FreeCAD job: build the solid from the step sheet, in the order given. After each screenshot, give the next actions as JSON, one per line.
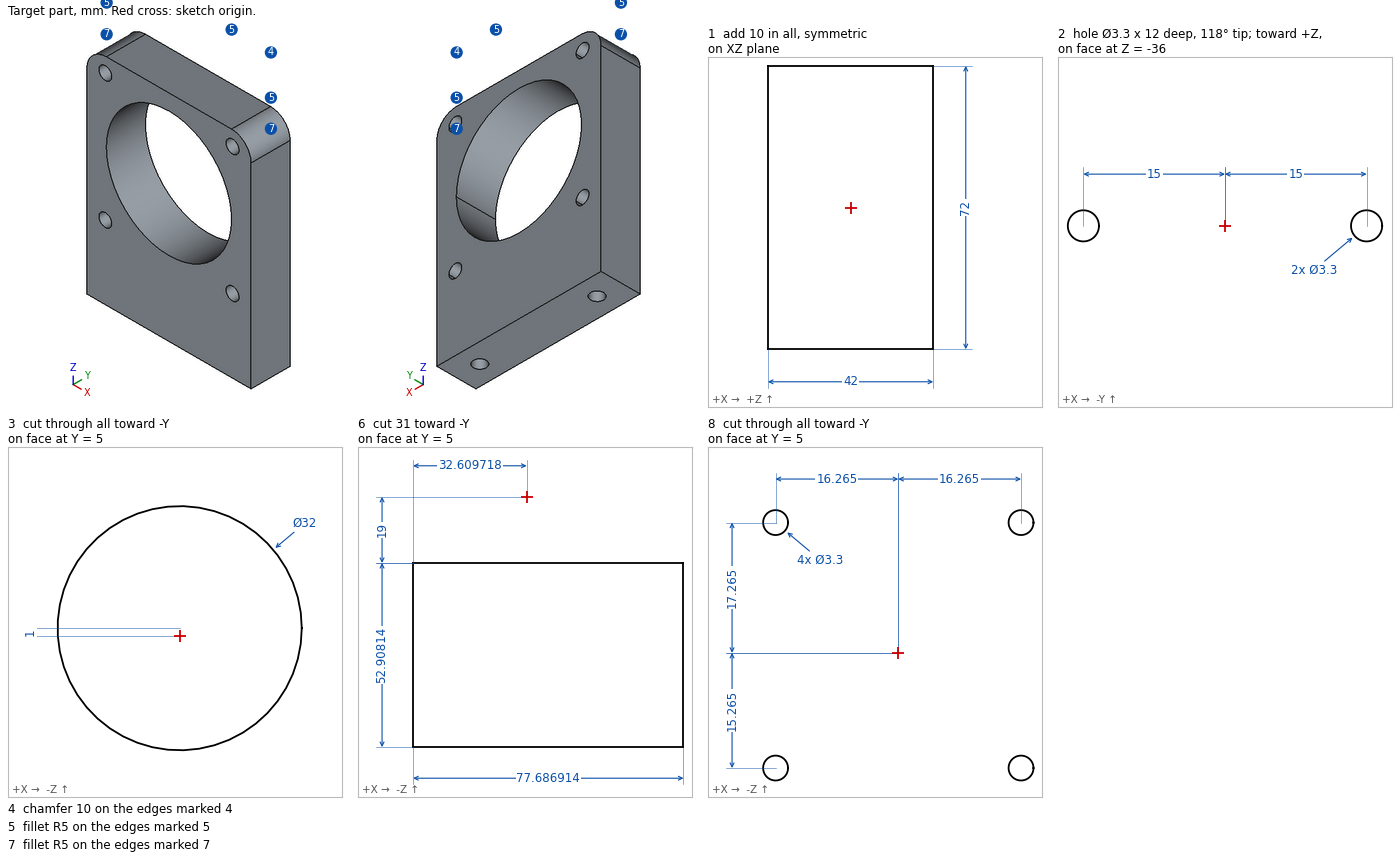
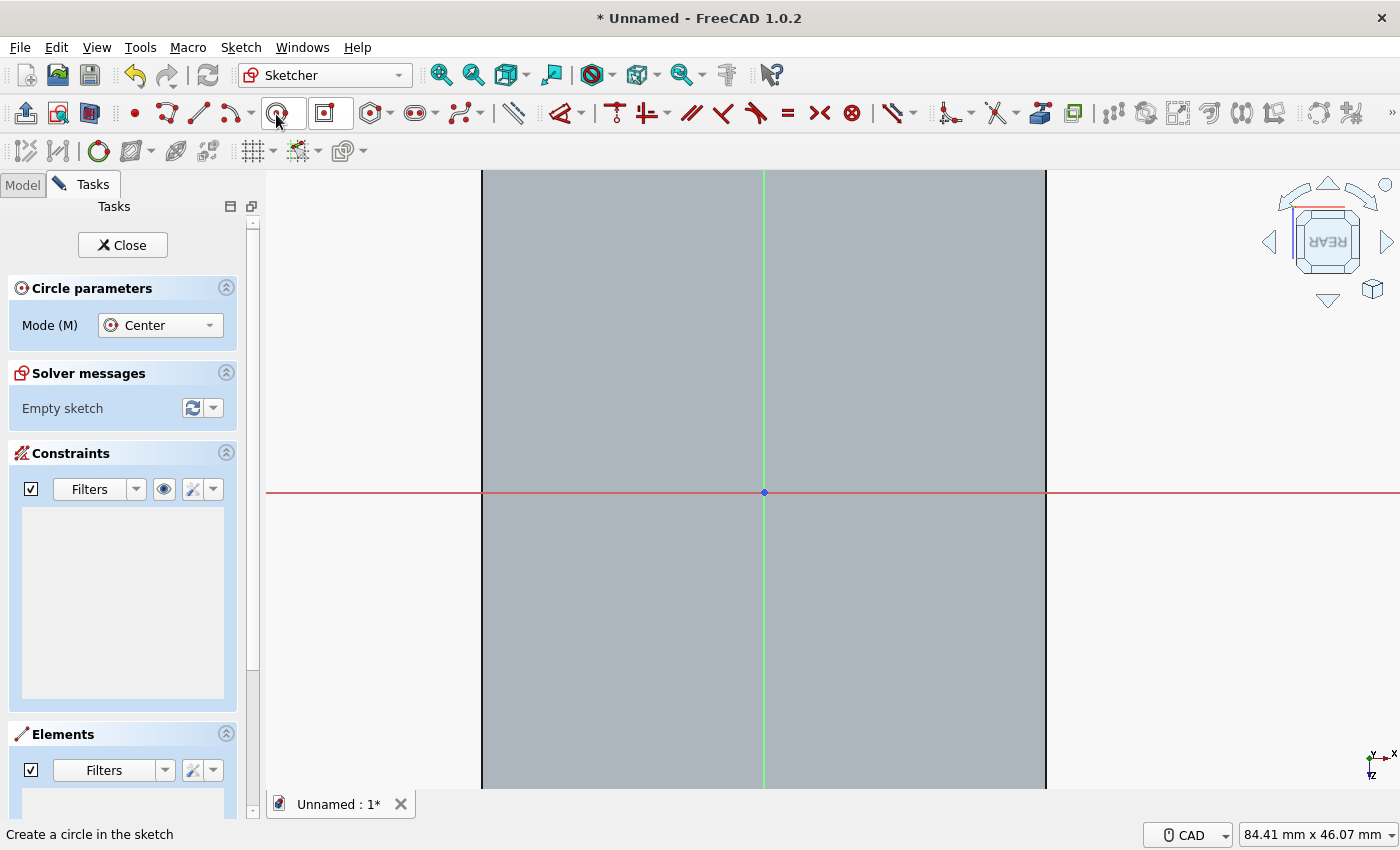
{"action": "left_click", "coordinate": [764, 479]}
{"action": "left_click", "coordinate": [916, 327]}
{"action": "key", "text": "Escape"}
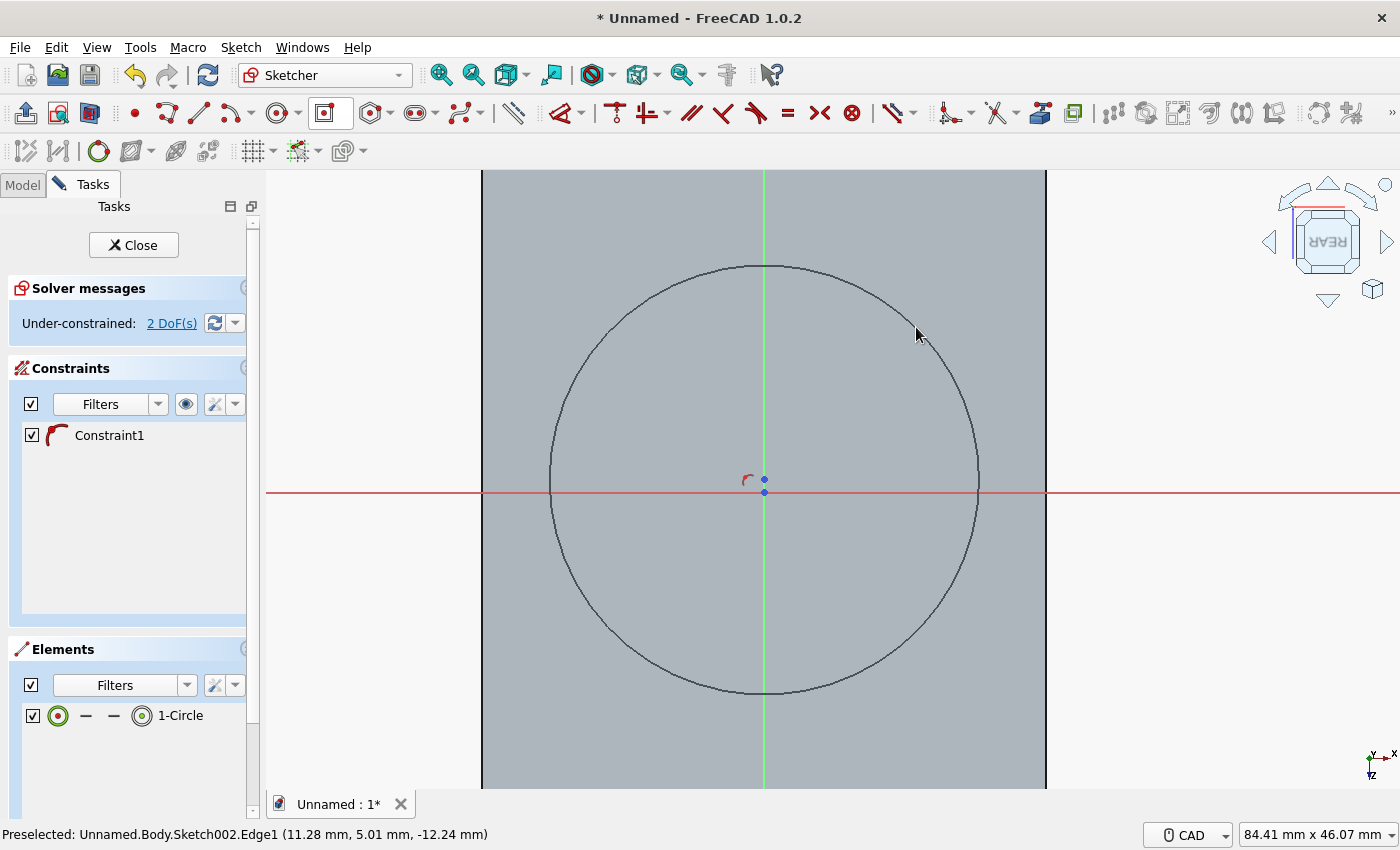
{"action": "left_click", "coordinate": [560, 114]}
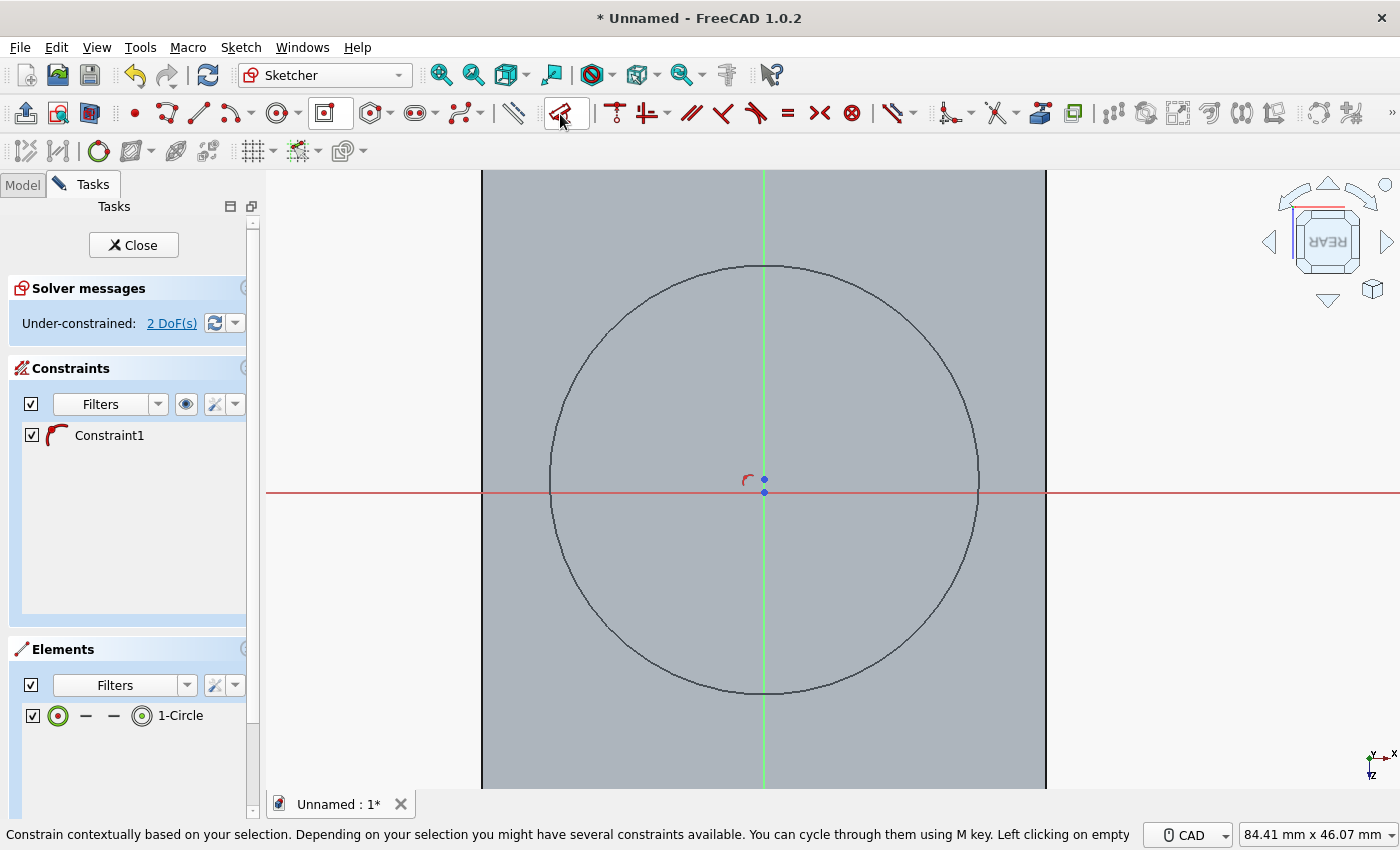
{"action": "left_click", "coordinate": [916, 328]}
{"action": "left_click", "coordinate": [939, 305]}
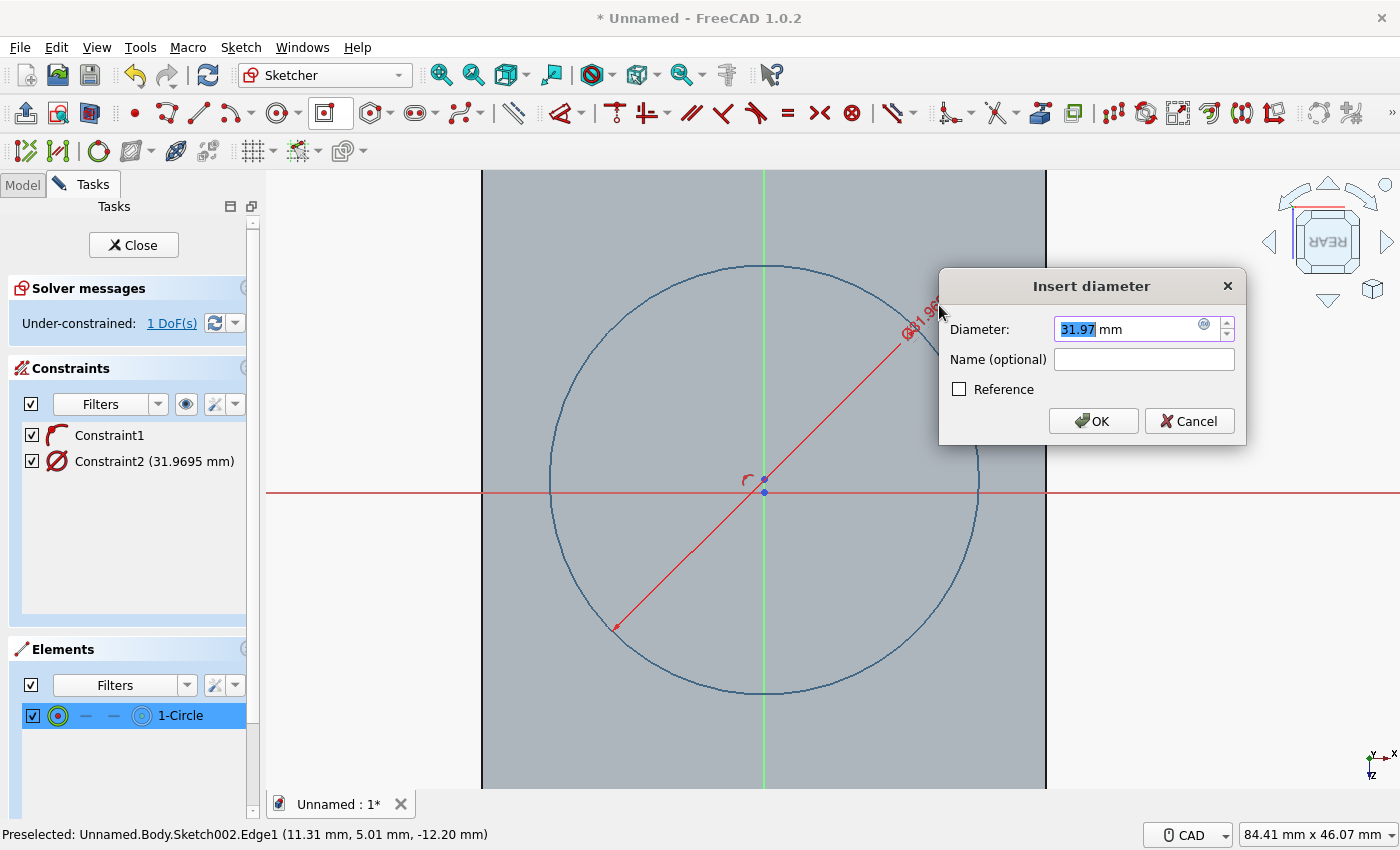
{"action": "type", "text": "32"}
{"action": "key", "text": "Return"}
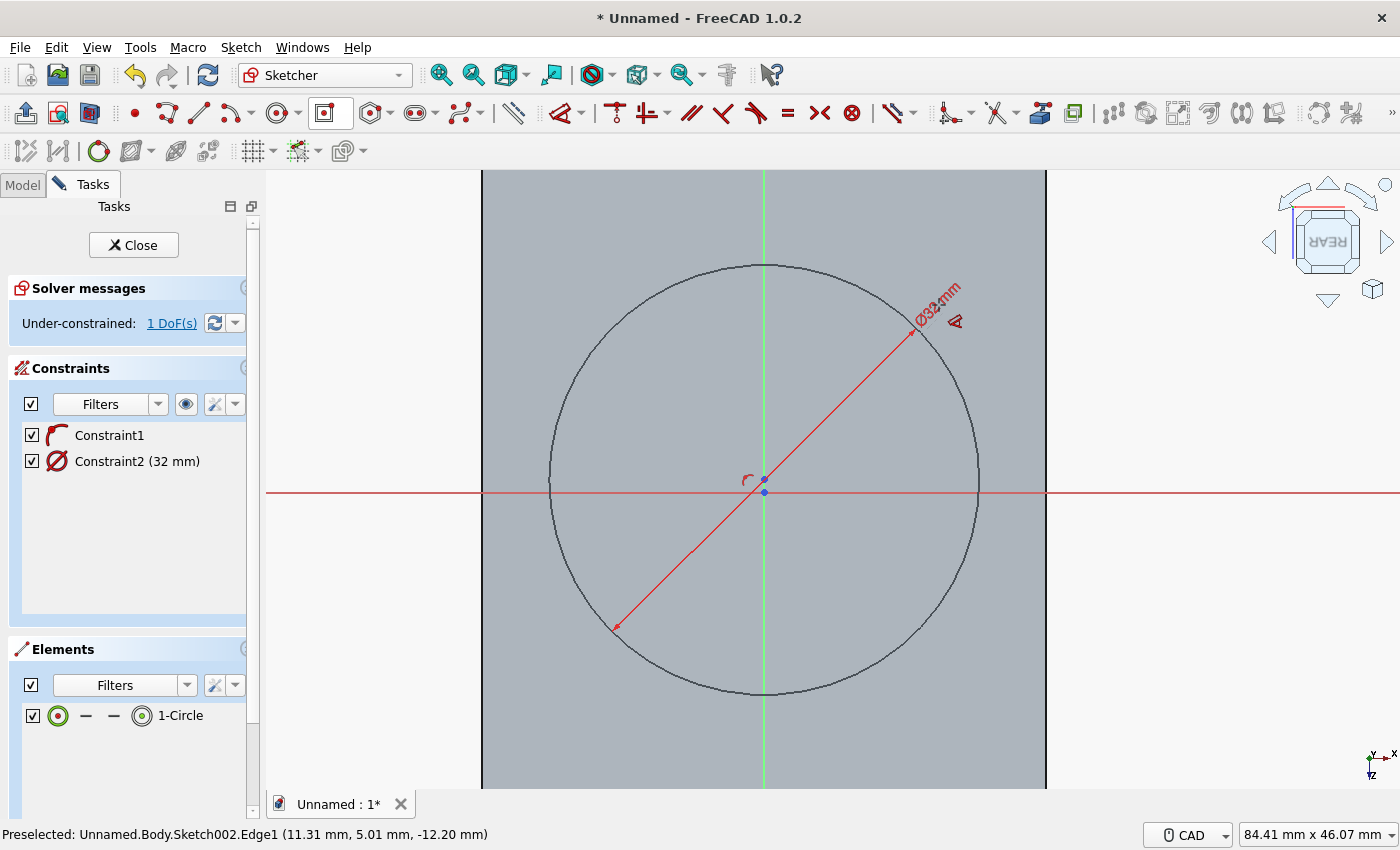
{"action": "scroll", "coordinate": [764, 480], "scroll_direction": "up", "scroll_amount": 6}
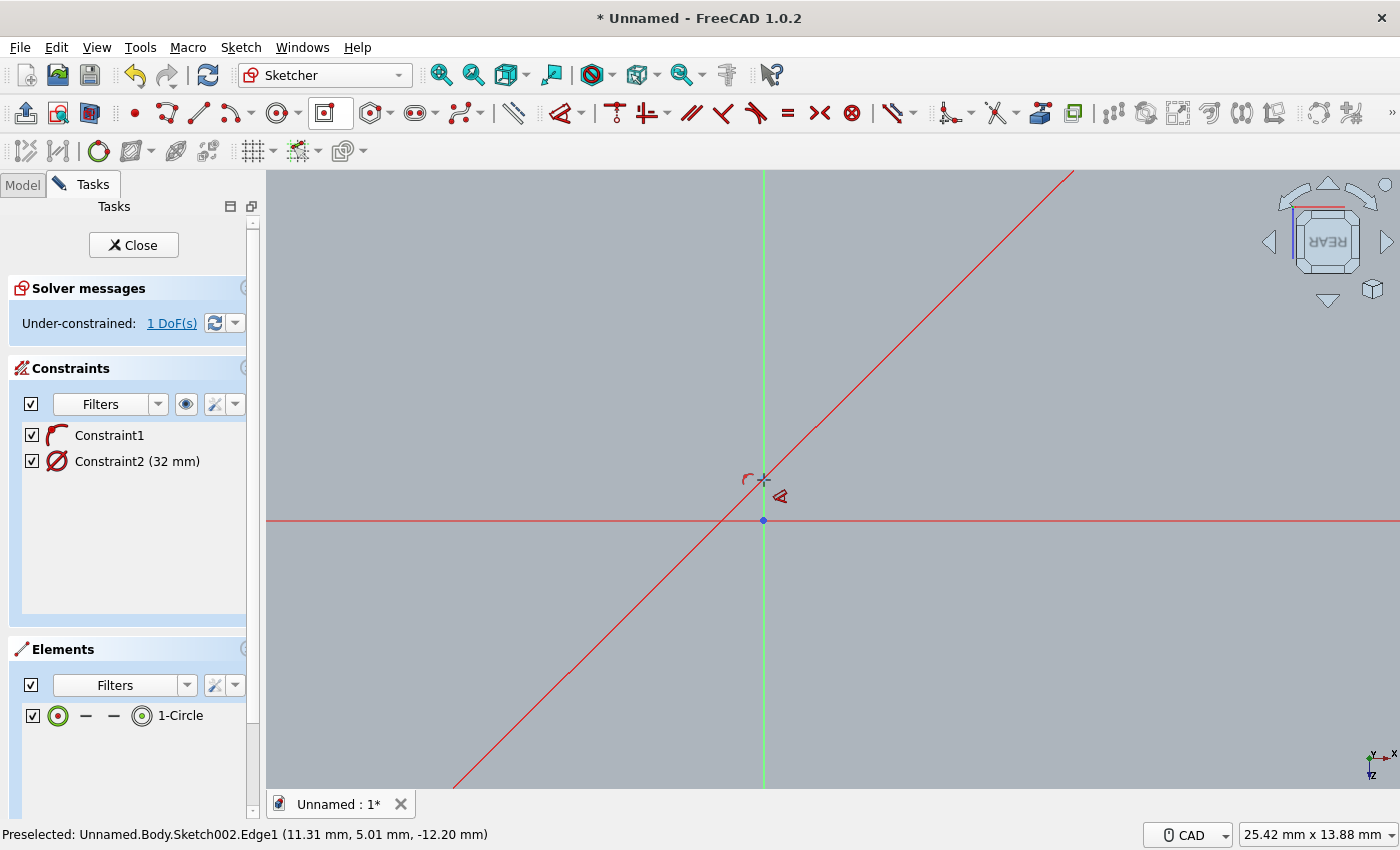
{"action": "left_click", "coordinate": [764, 479]}
{"action": "left_click", "coordinate": [798, 500]}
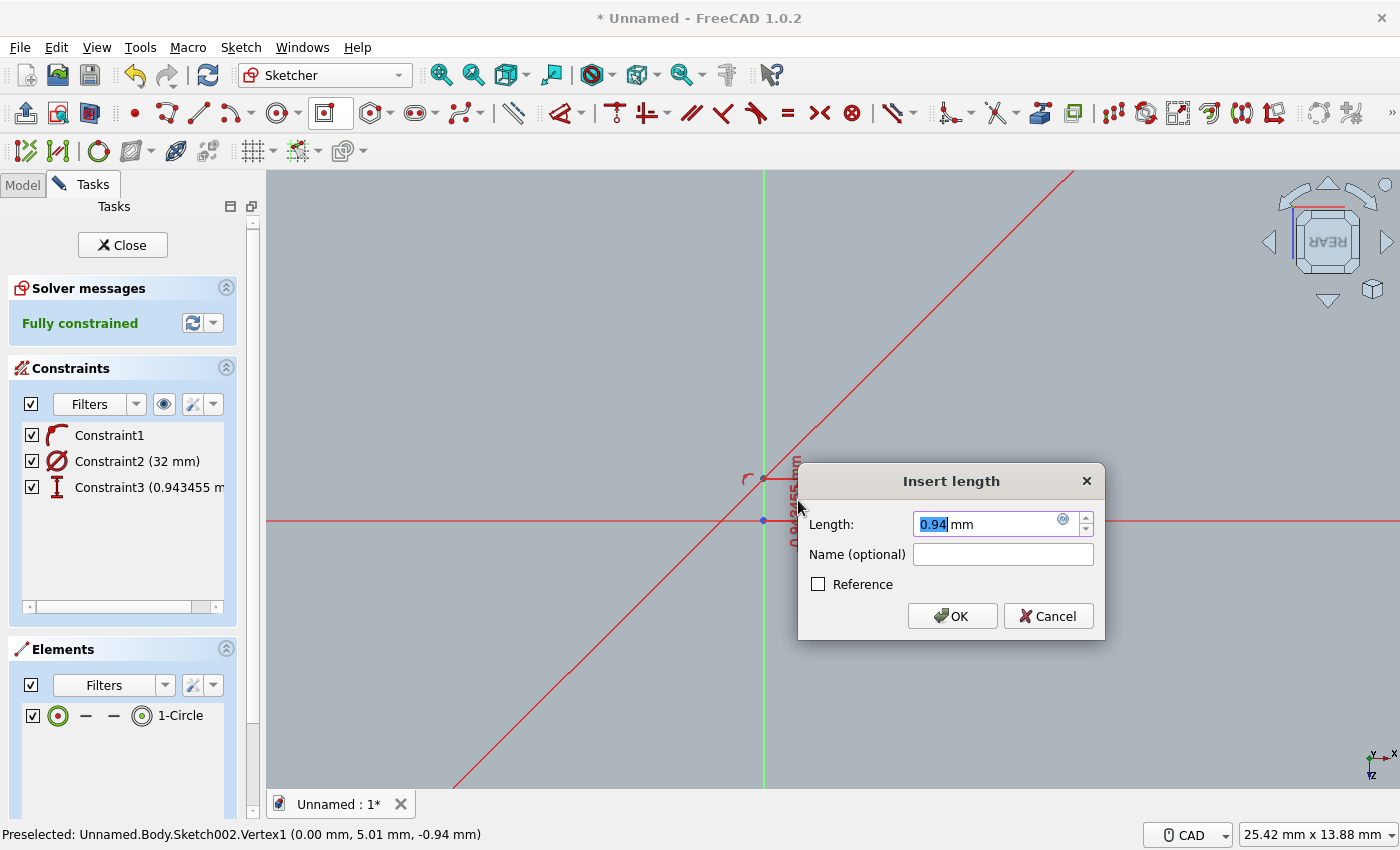
{"action": "type", "text": "1"}
{"action": "key", "text": "Return"}
{"action": "key", "text": "Escape"}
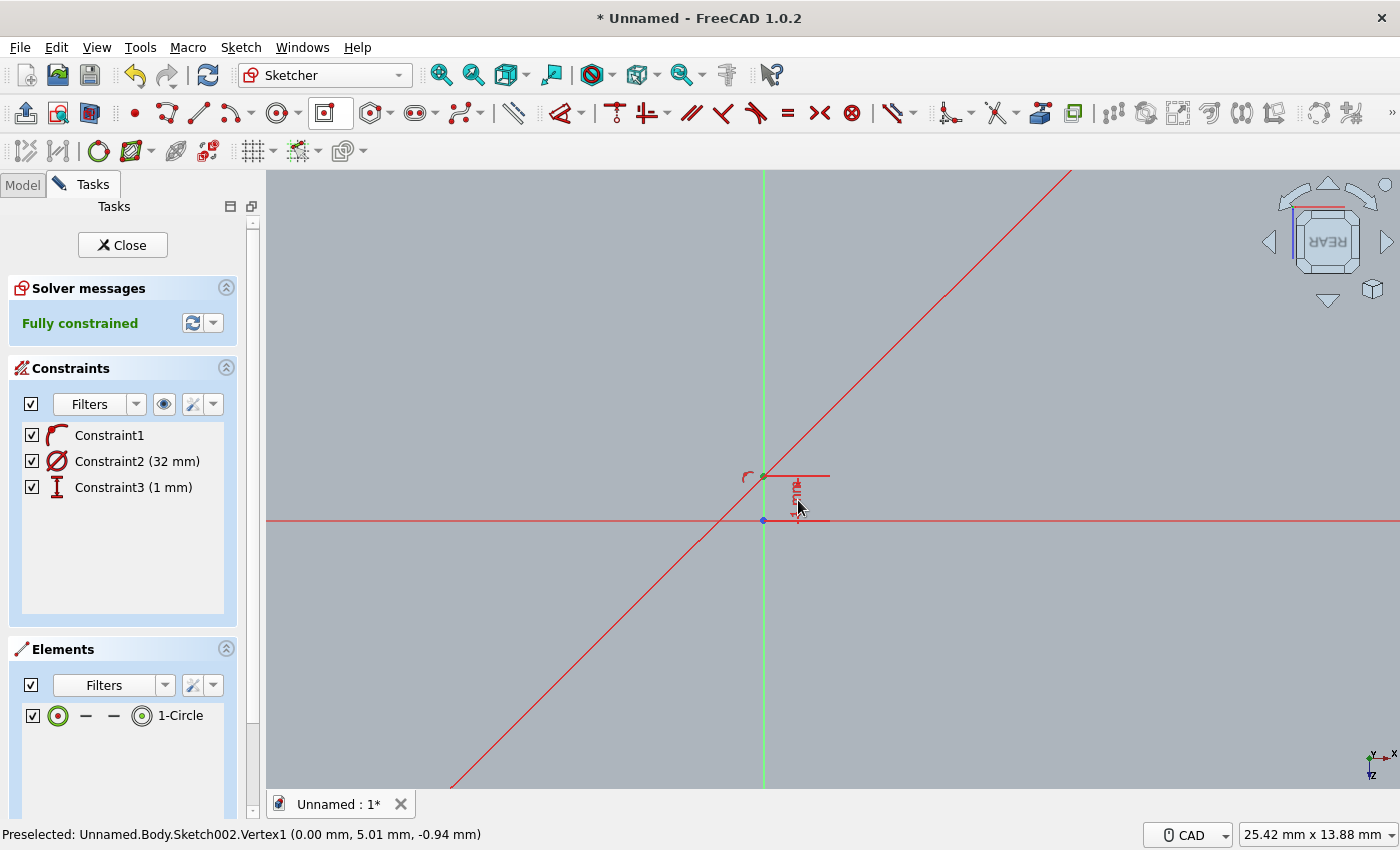
{"action": "left_click", "coordinate": [123, 245]}